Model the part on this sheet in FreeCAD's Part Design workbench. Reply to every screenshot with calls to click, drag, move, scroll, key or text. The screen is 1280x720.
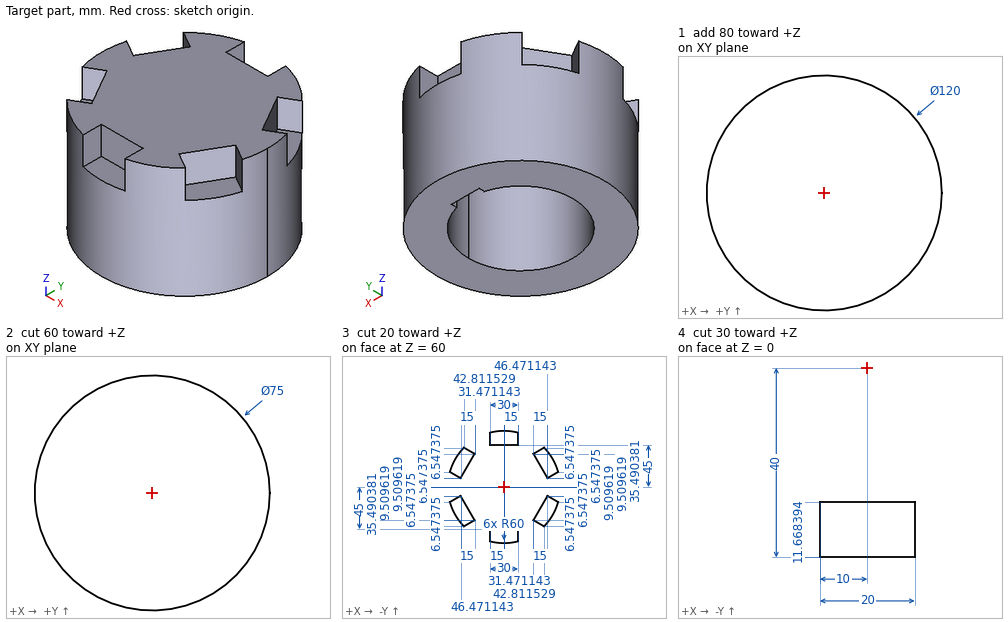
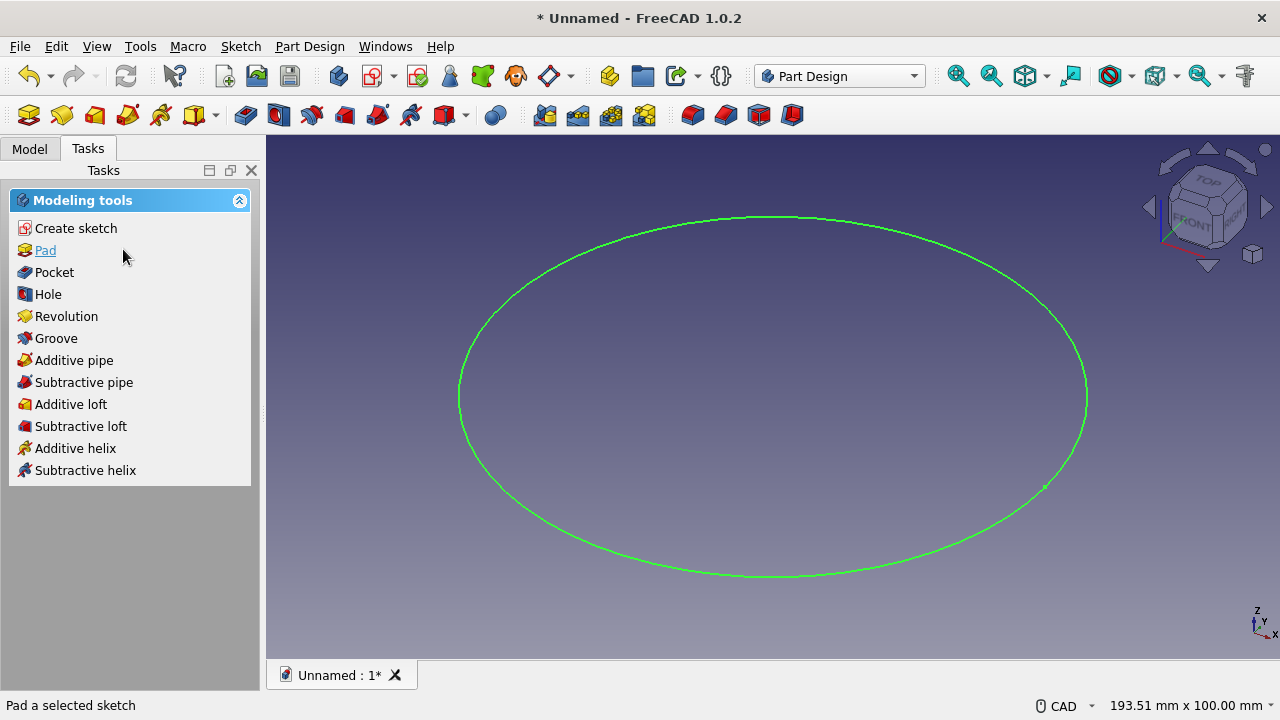
click(29, 116)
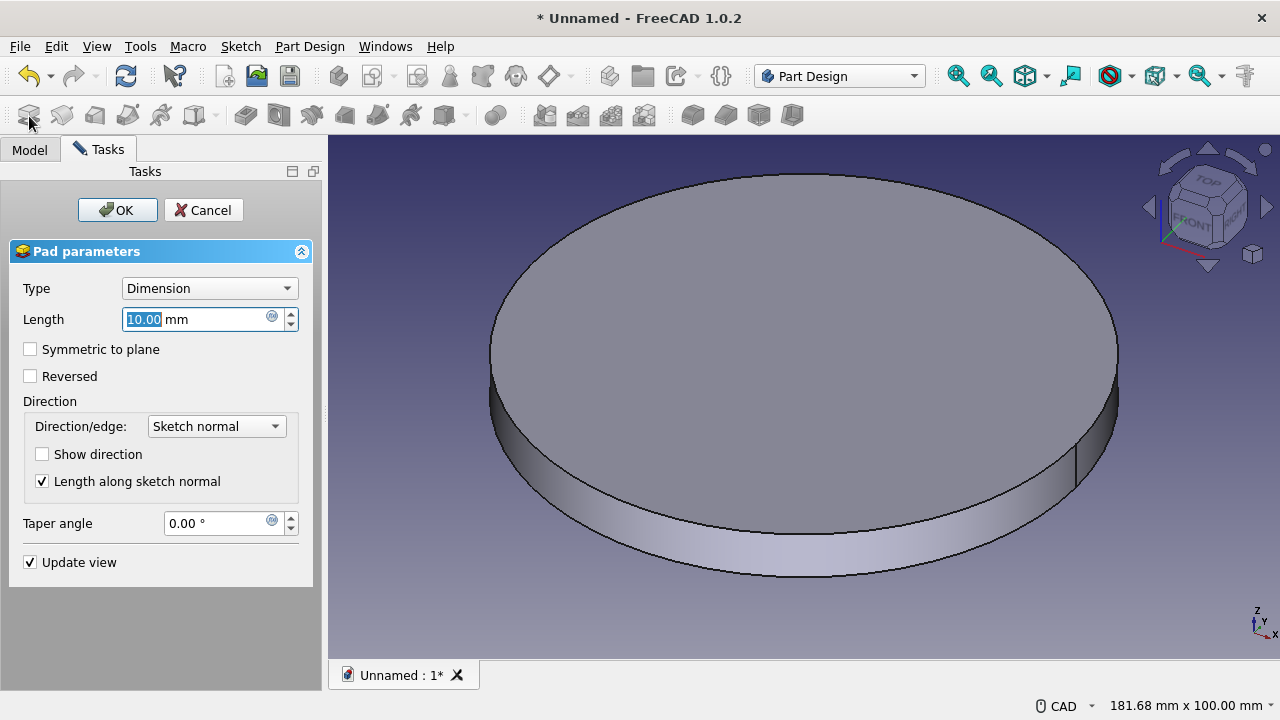
text(80)
key(Tab)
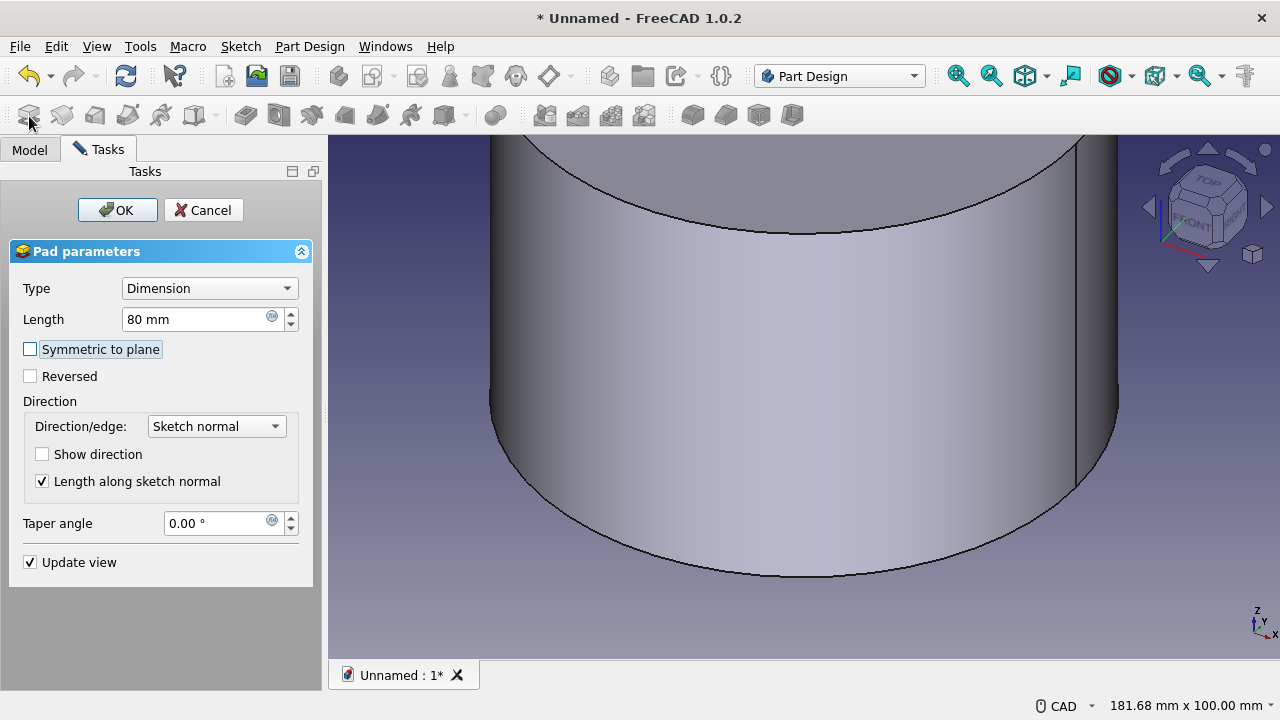
click(118, 210)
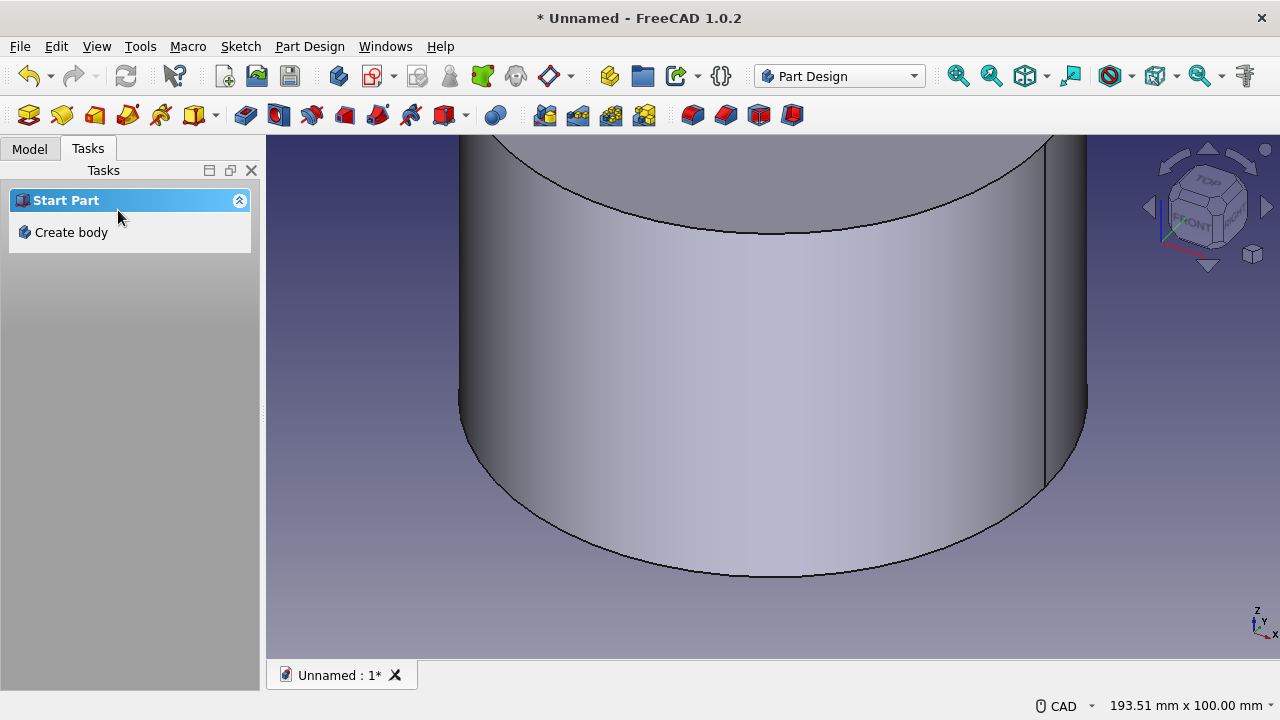
click(959, 76)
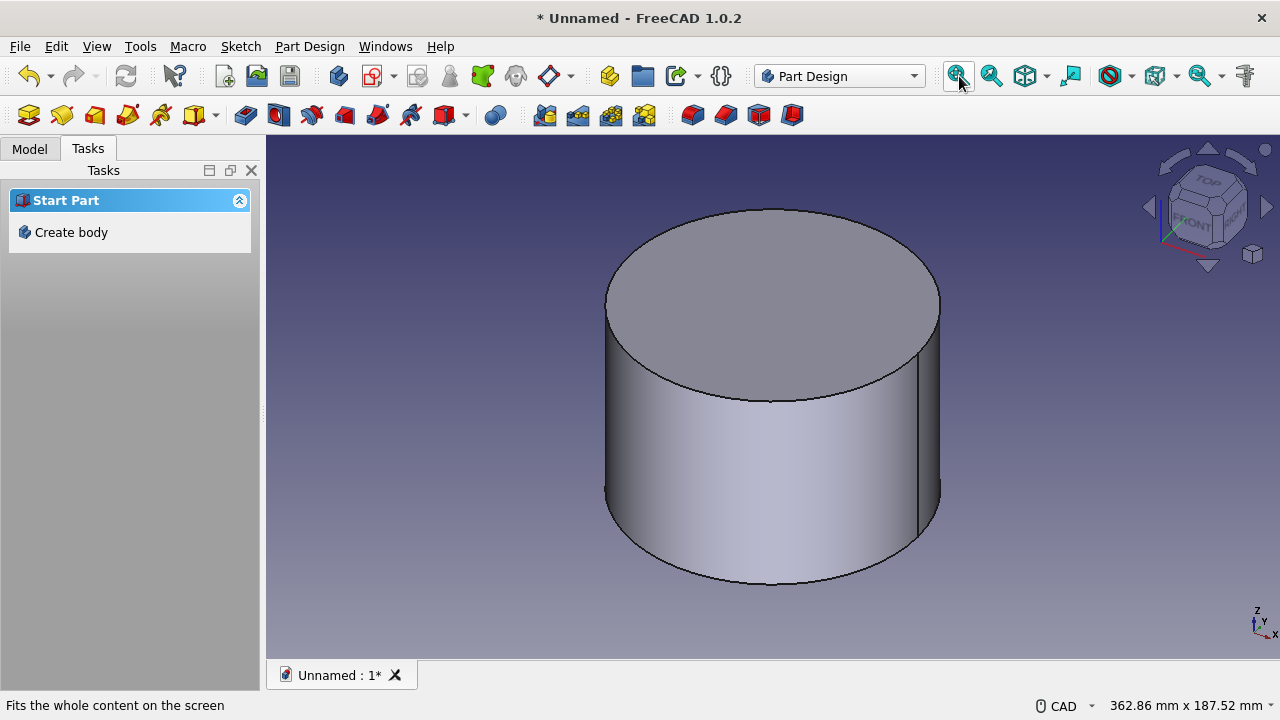
click(372, 76)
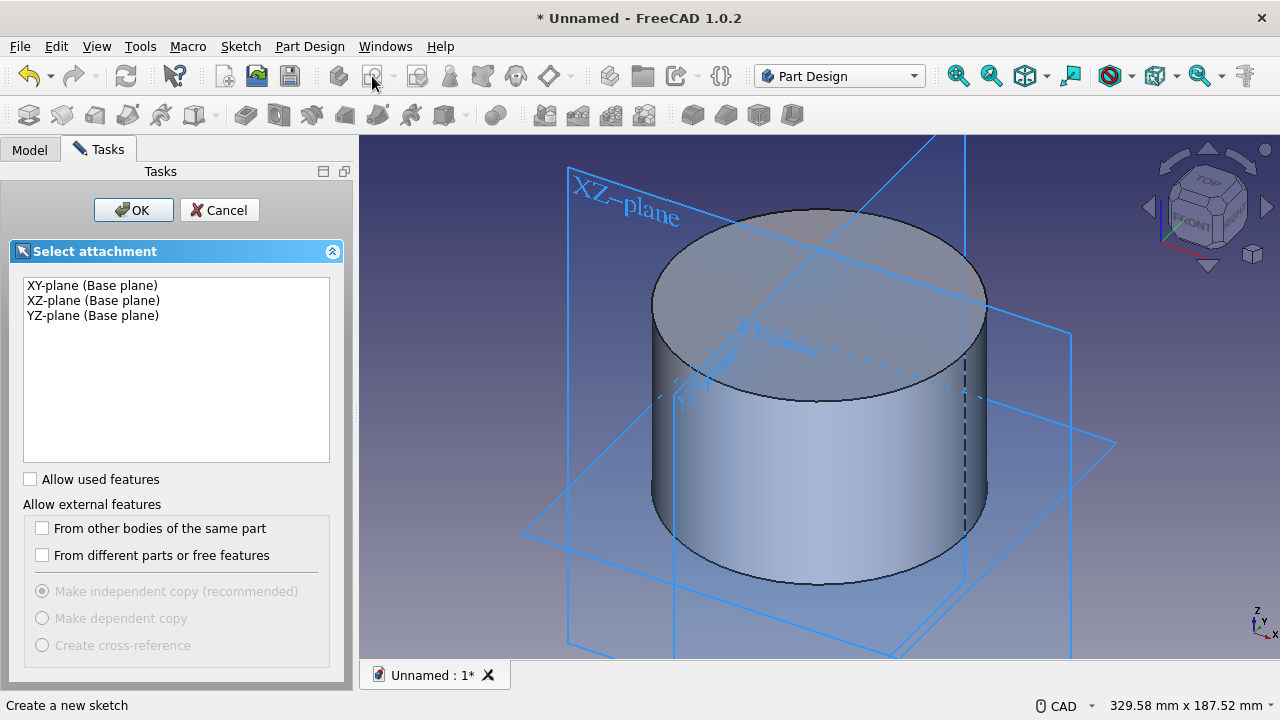
click(84, 286)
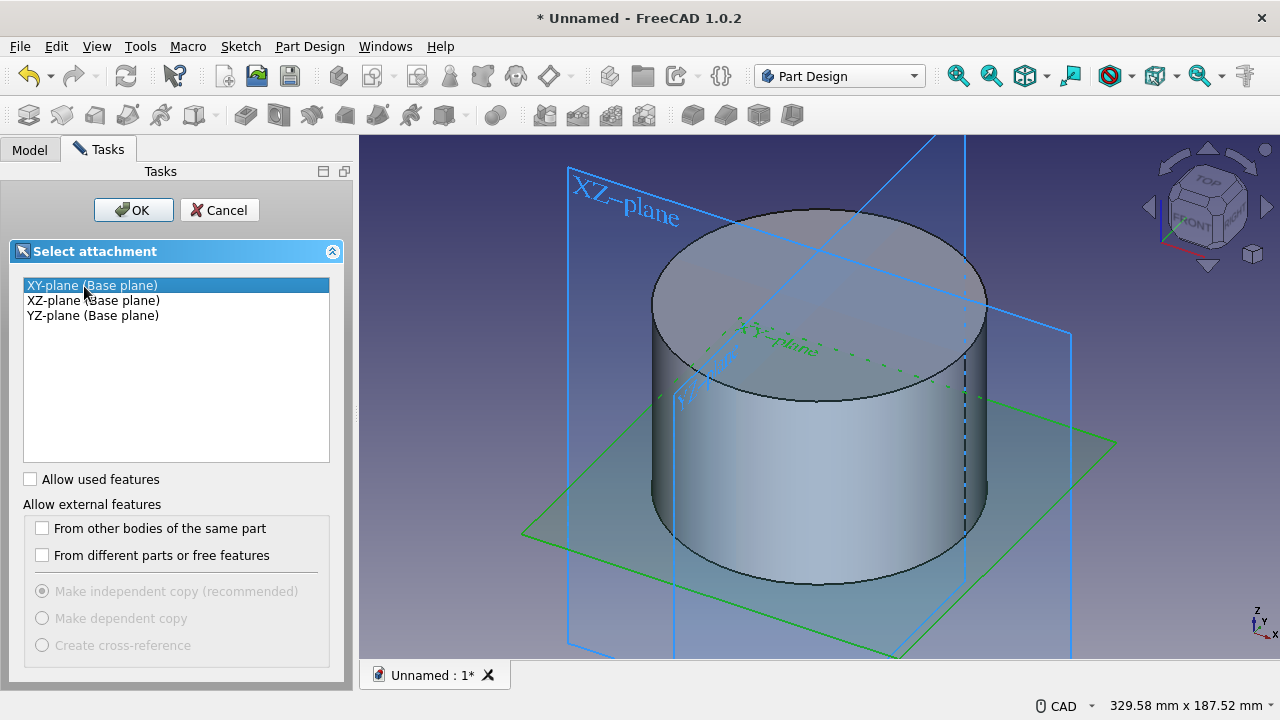
click(134, 210)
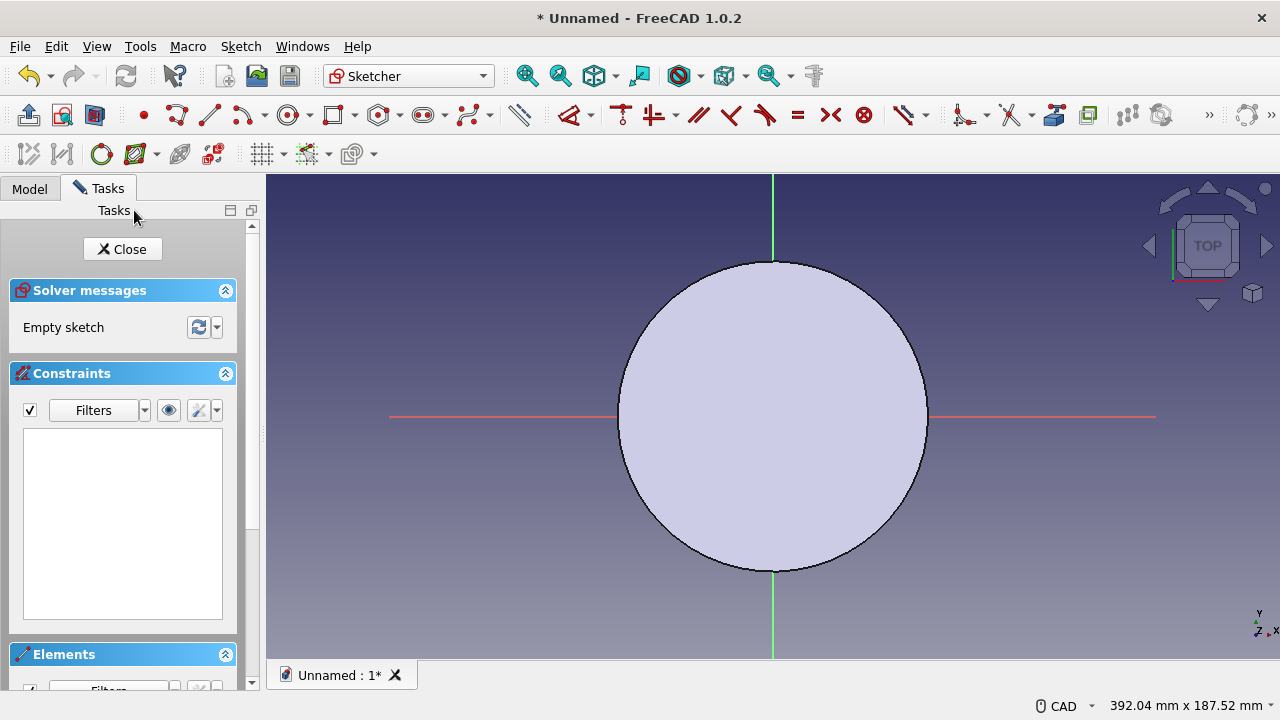
click(95, 116)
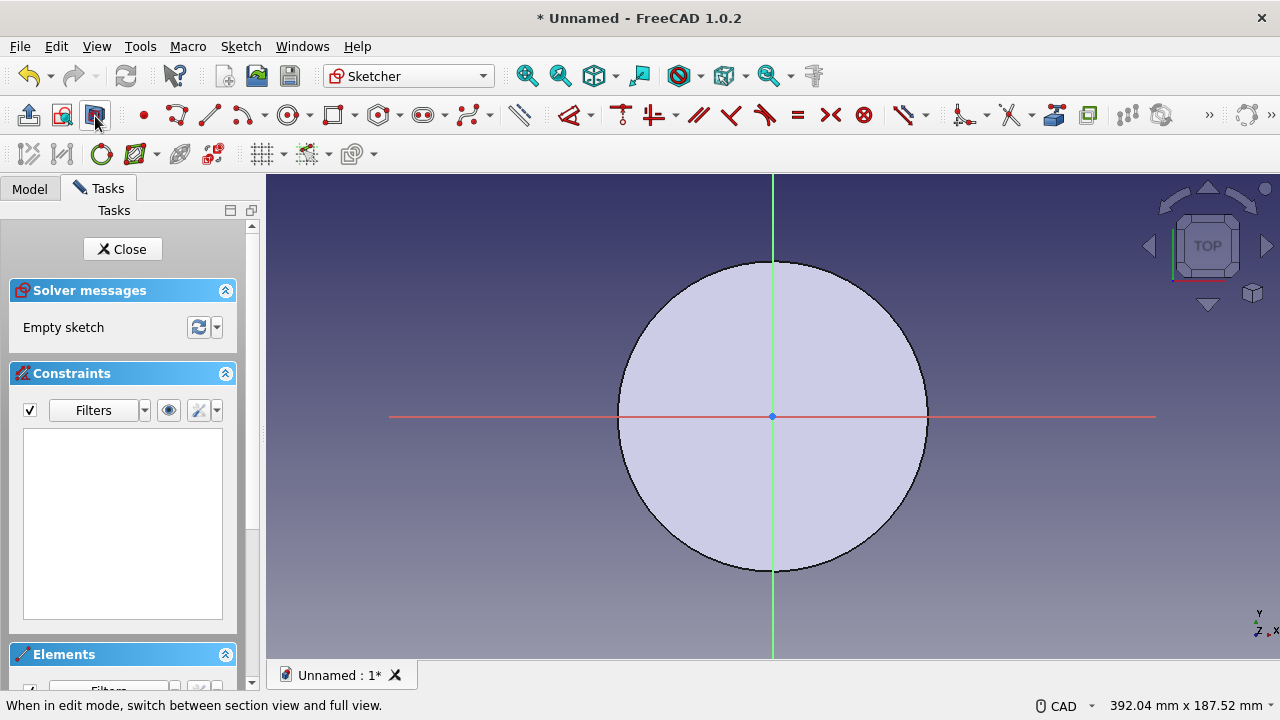
scroll(912, 416, up, 2)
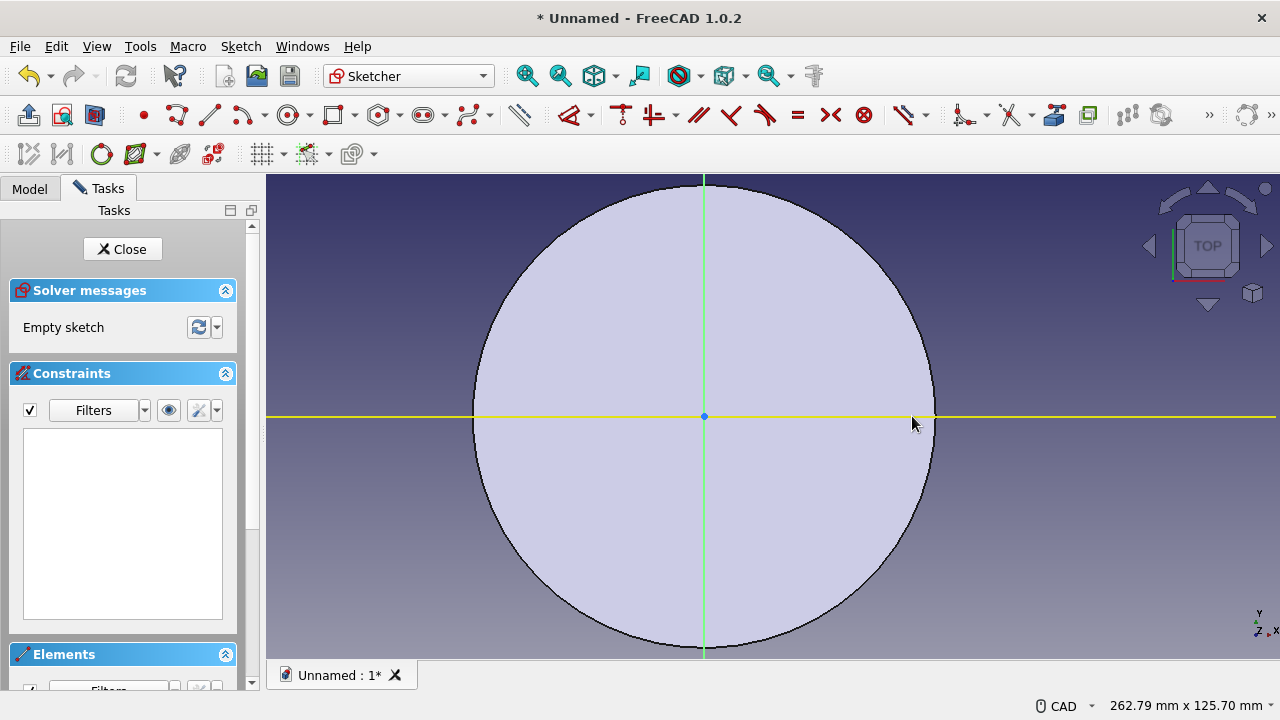
click(288, 116)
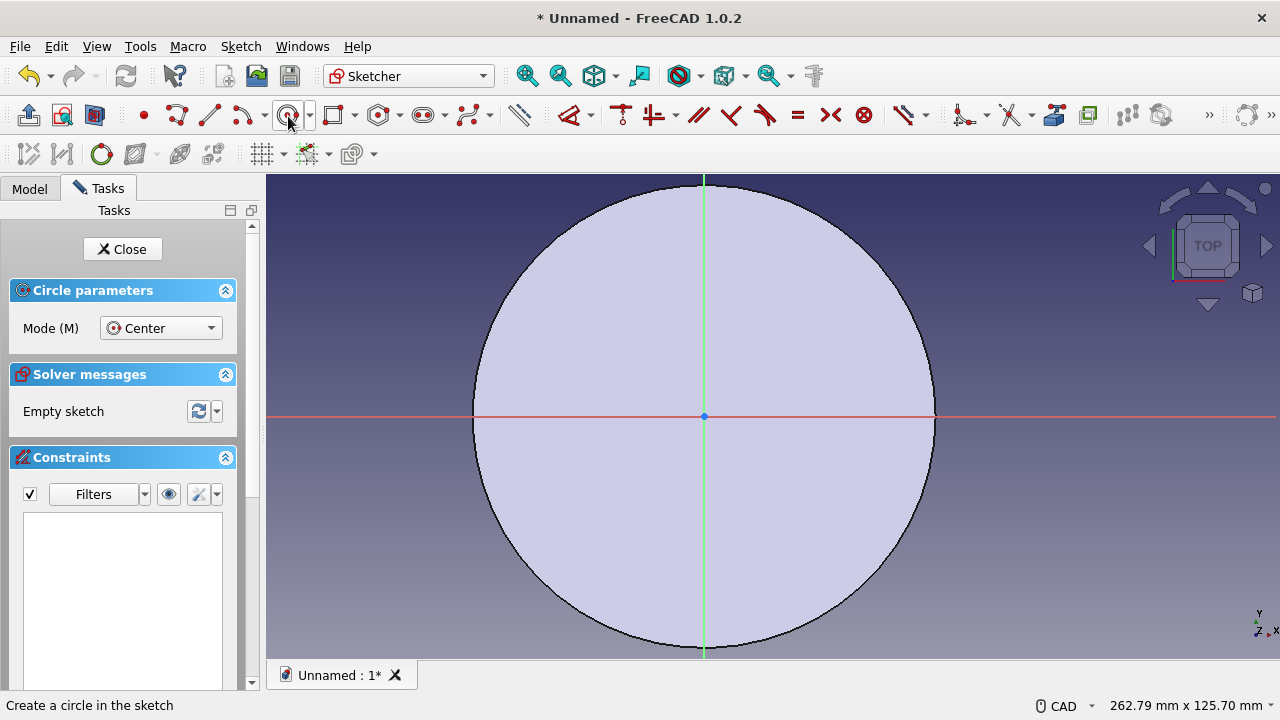
click(704, 416)
click(806, 314)
key(Escape)